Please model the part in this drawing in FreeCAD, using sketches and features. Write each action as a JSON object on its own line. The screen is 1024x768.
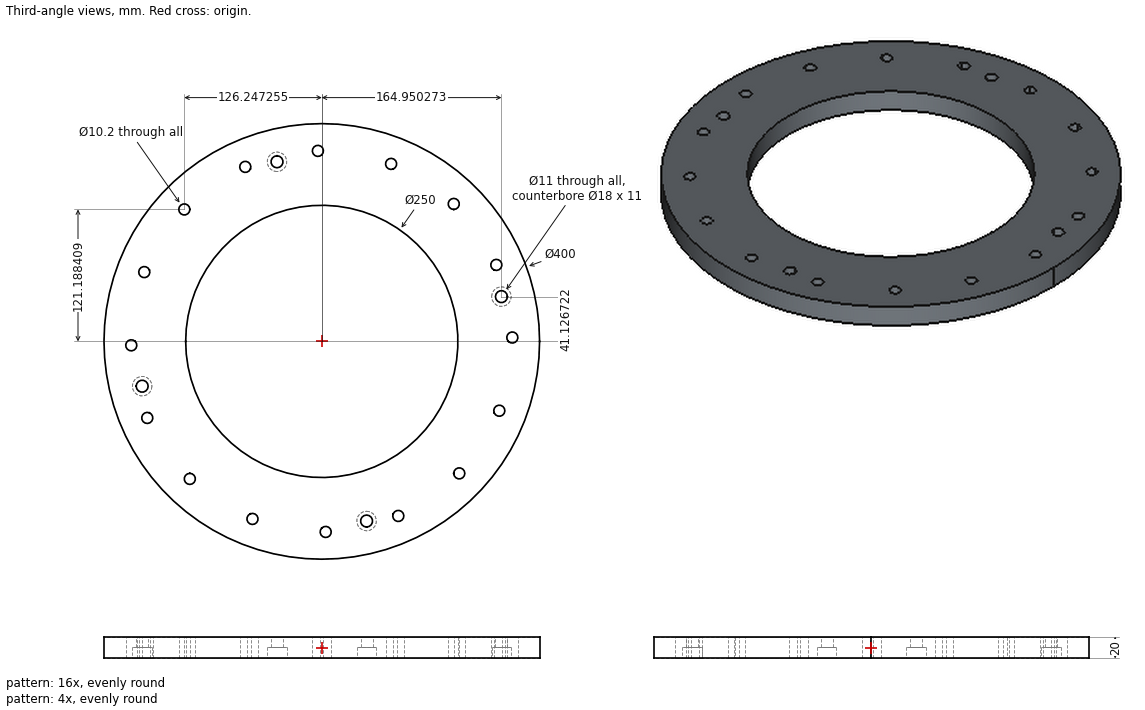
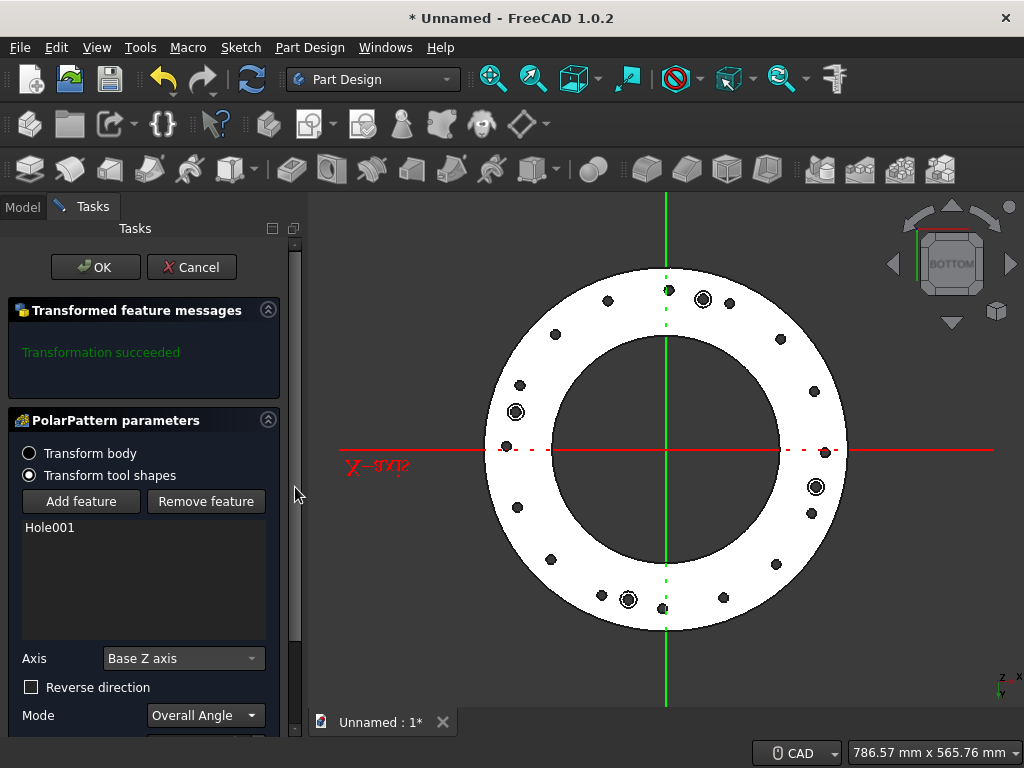
{"action": "left_click", "coordinate": [96, 267]}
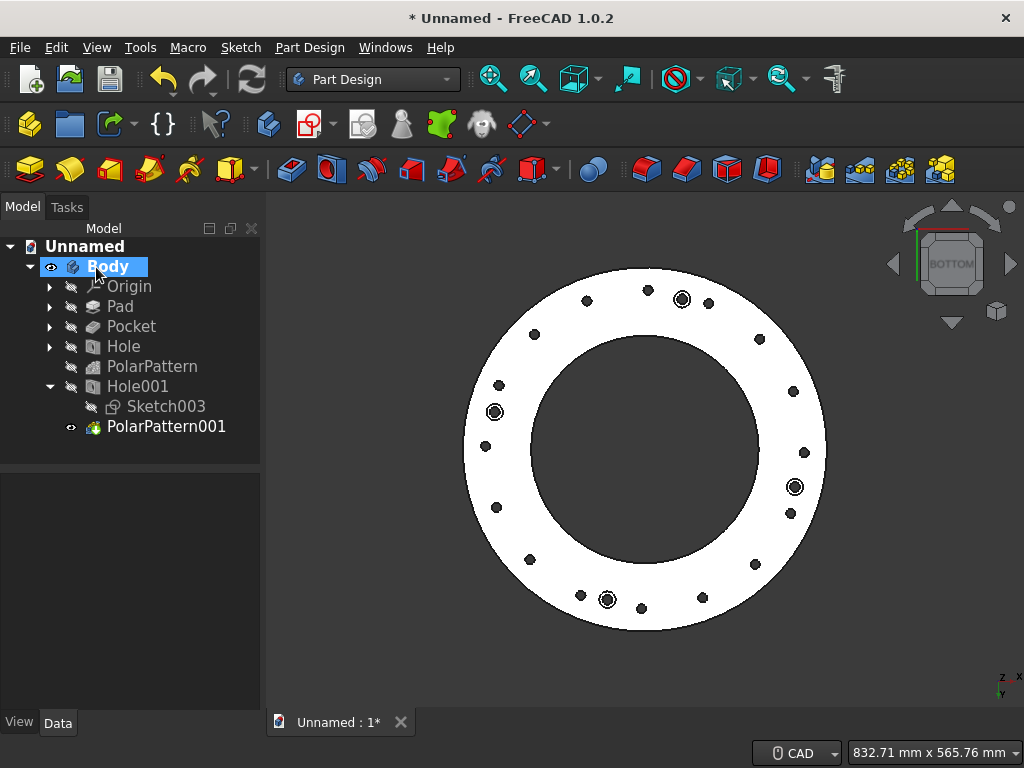
{"action": "key", "text": "0"}